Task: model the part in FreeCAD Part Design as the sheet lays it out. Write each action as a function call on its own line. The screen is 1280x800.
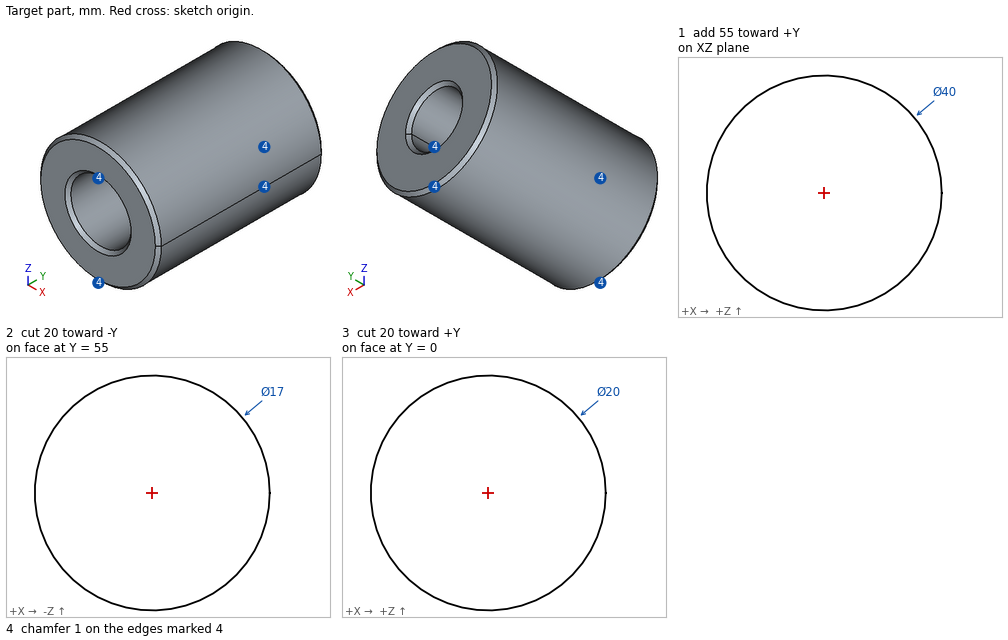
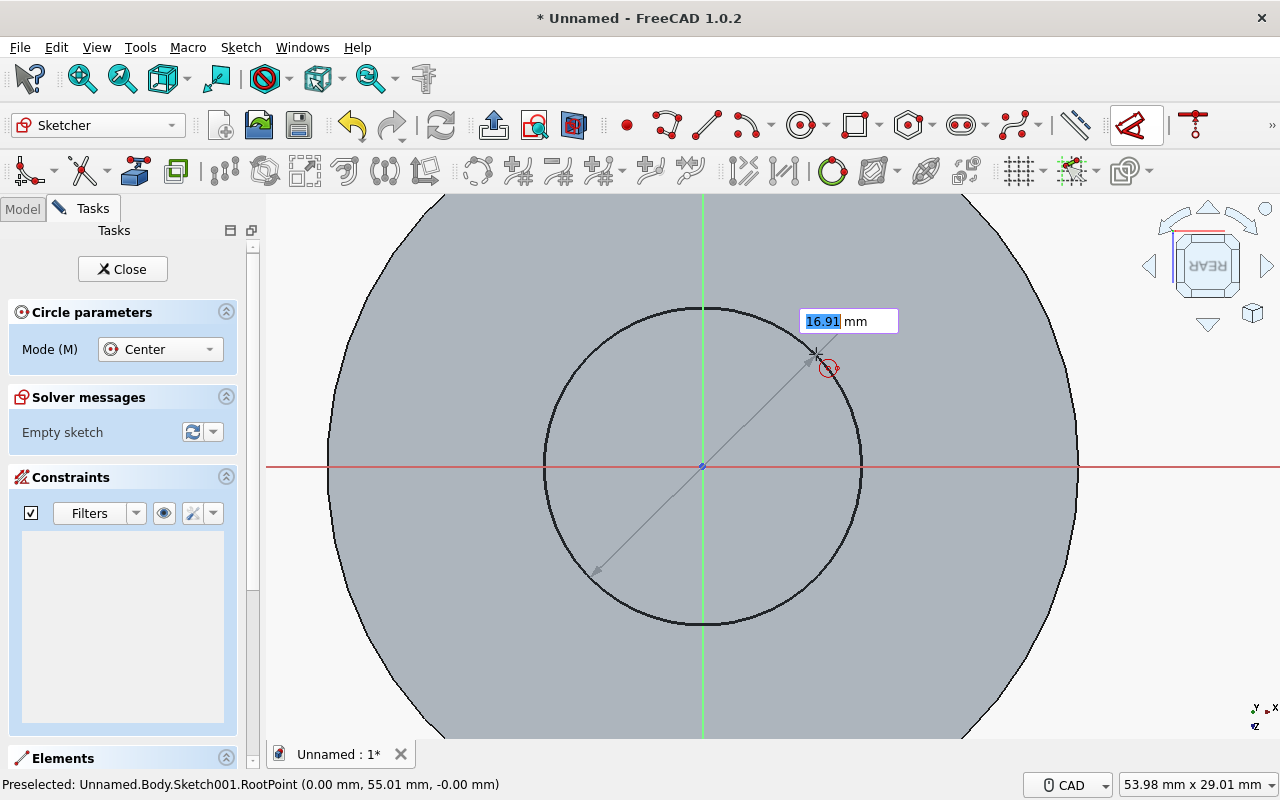
text(17)
key(Return)
key(Escape)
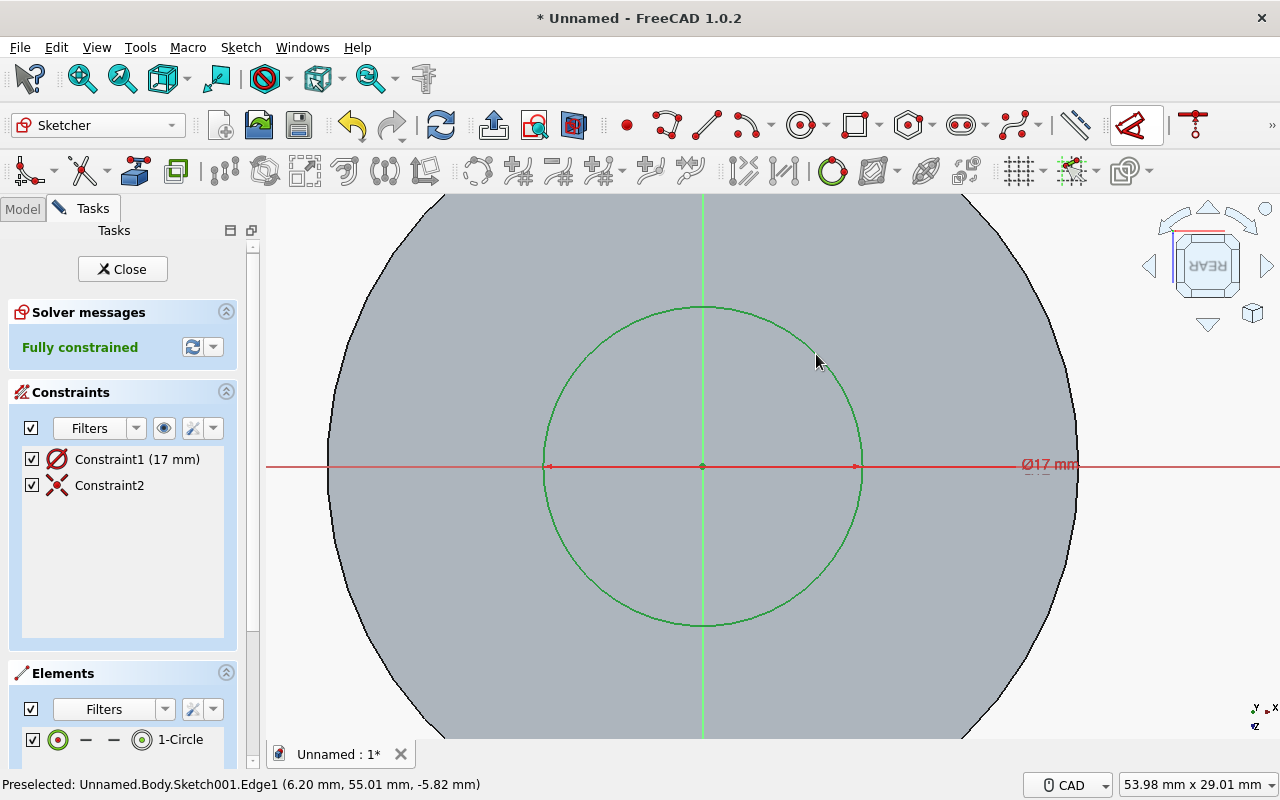
click(123, 269)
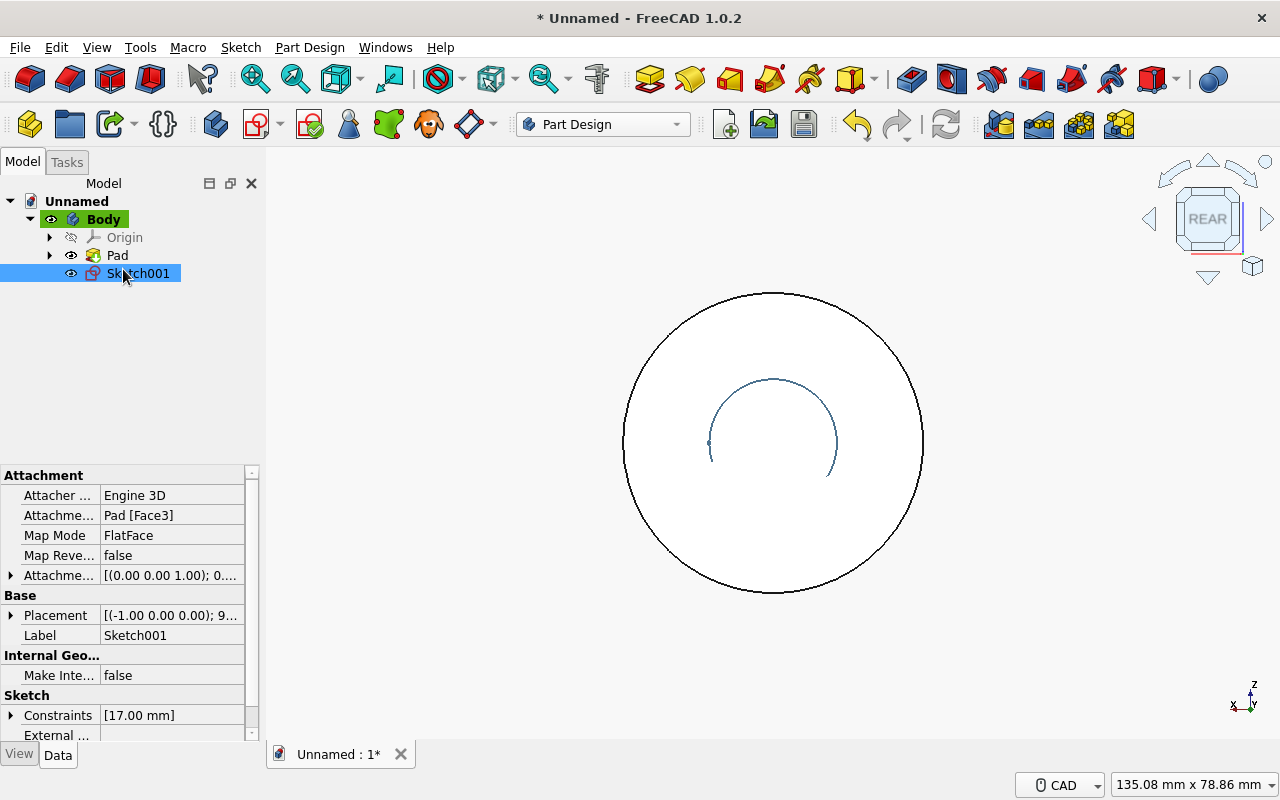
click(912, 80)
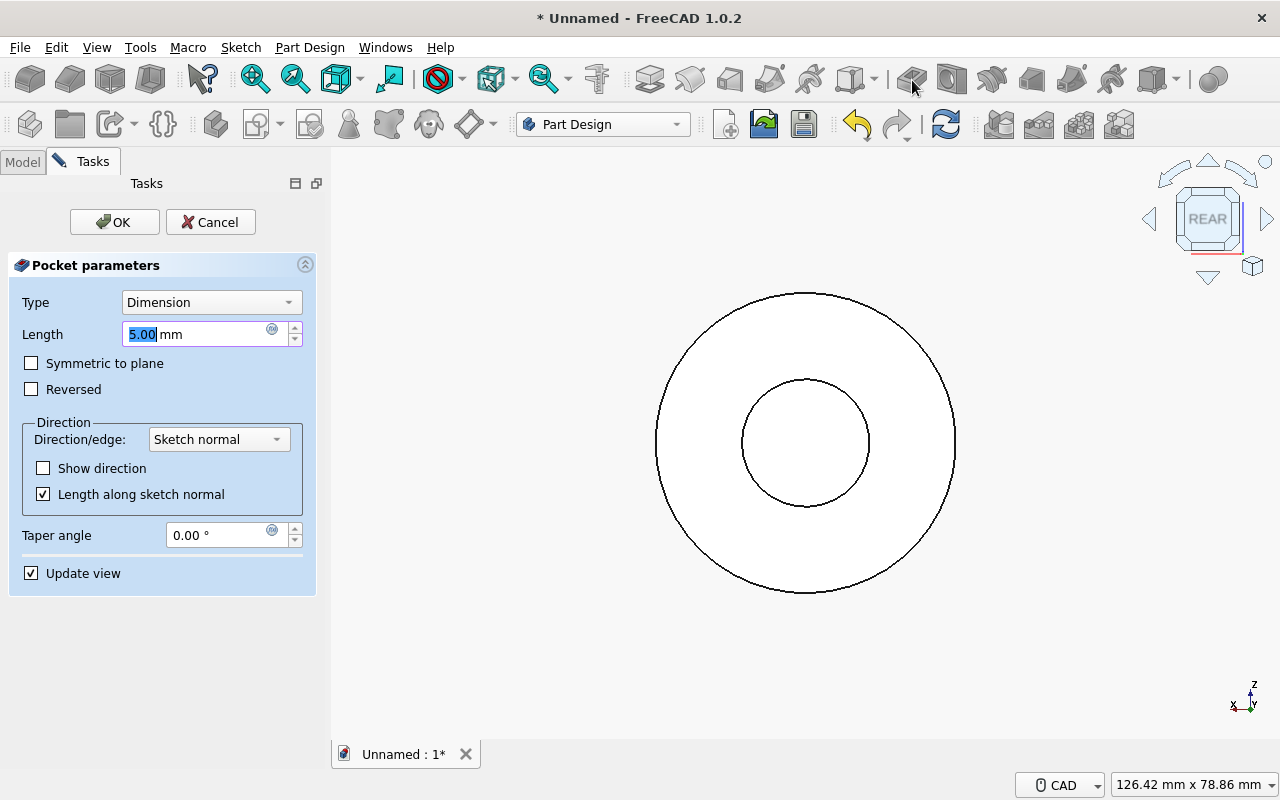
text(20)
key(Tab)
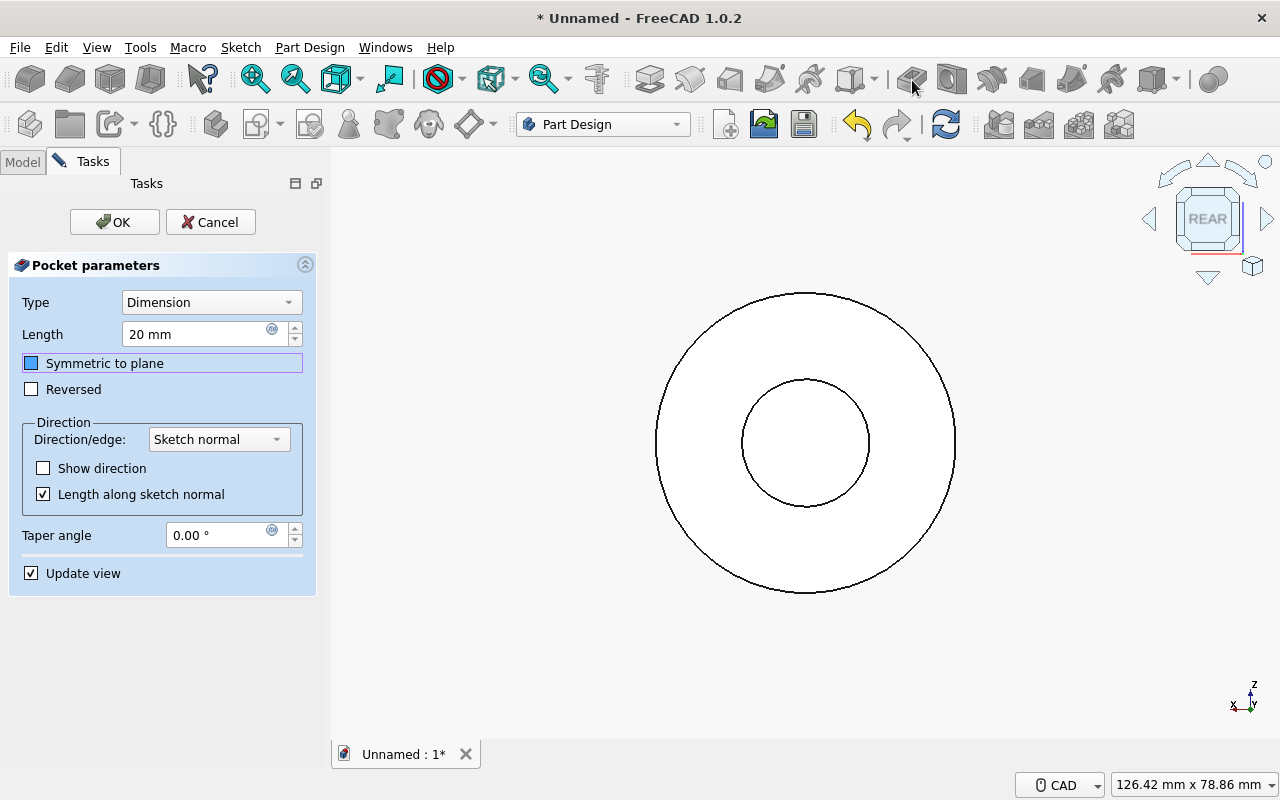
click(115, 222)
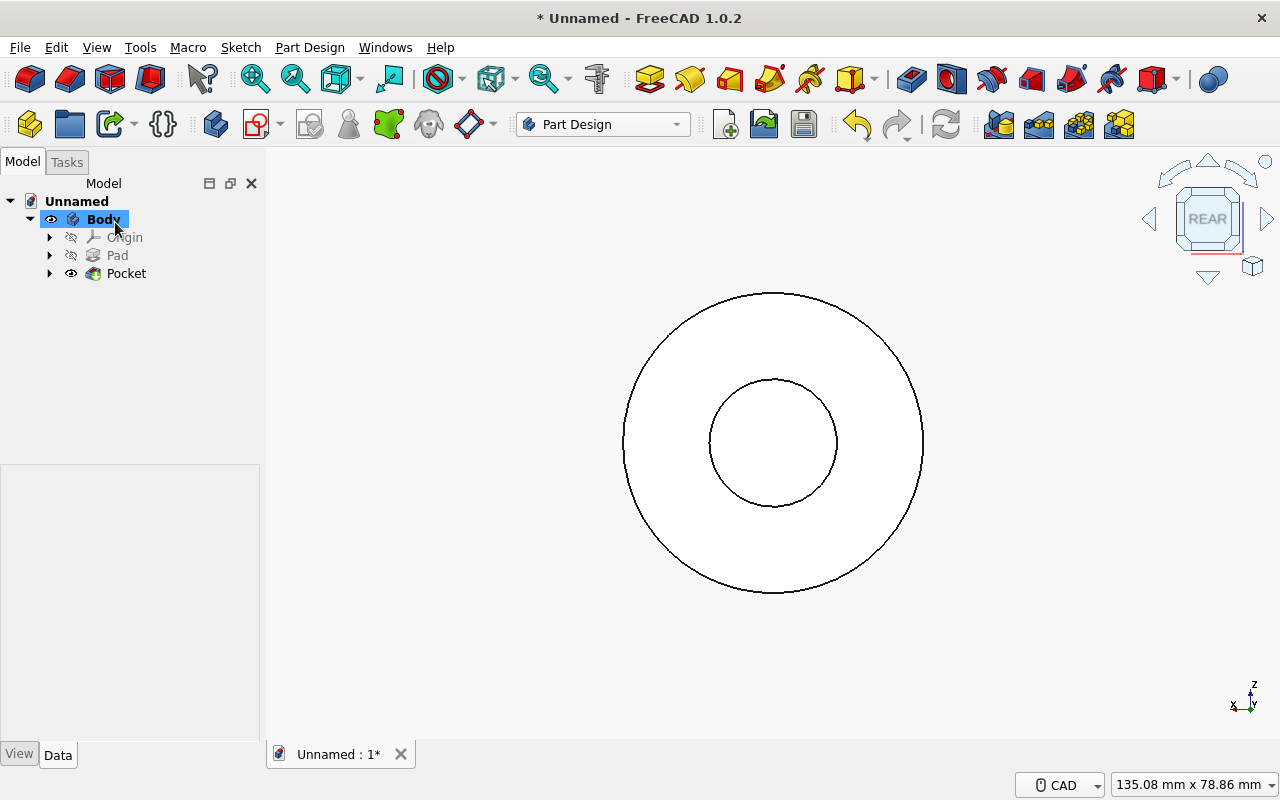
key(0)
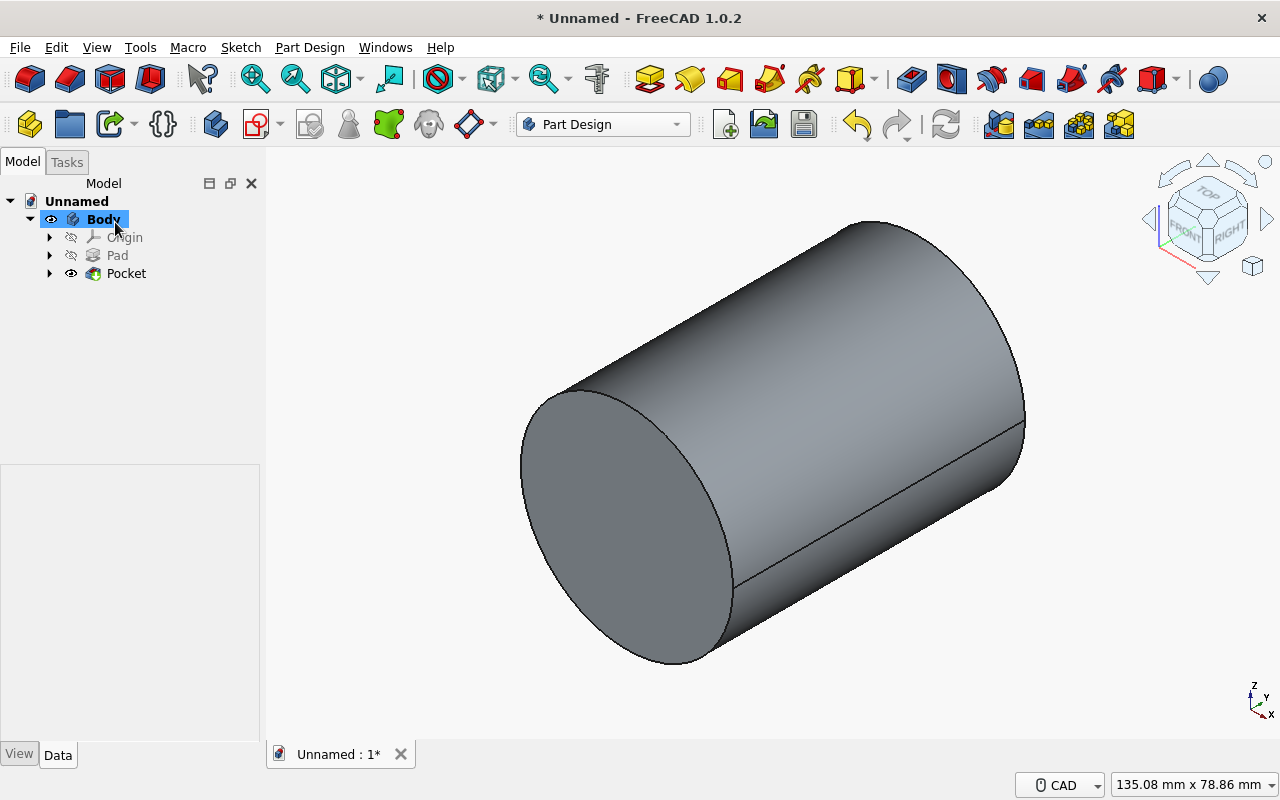
click(627, 526)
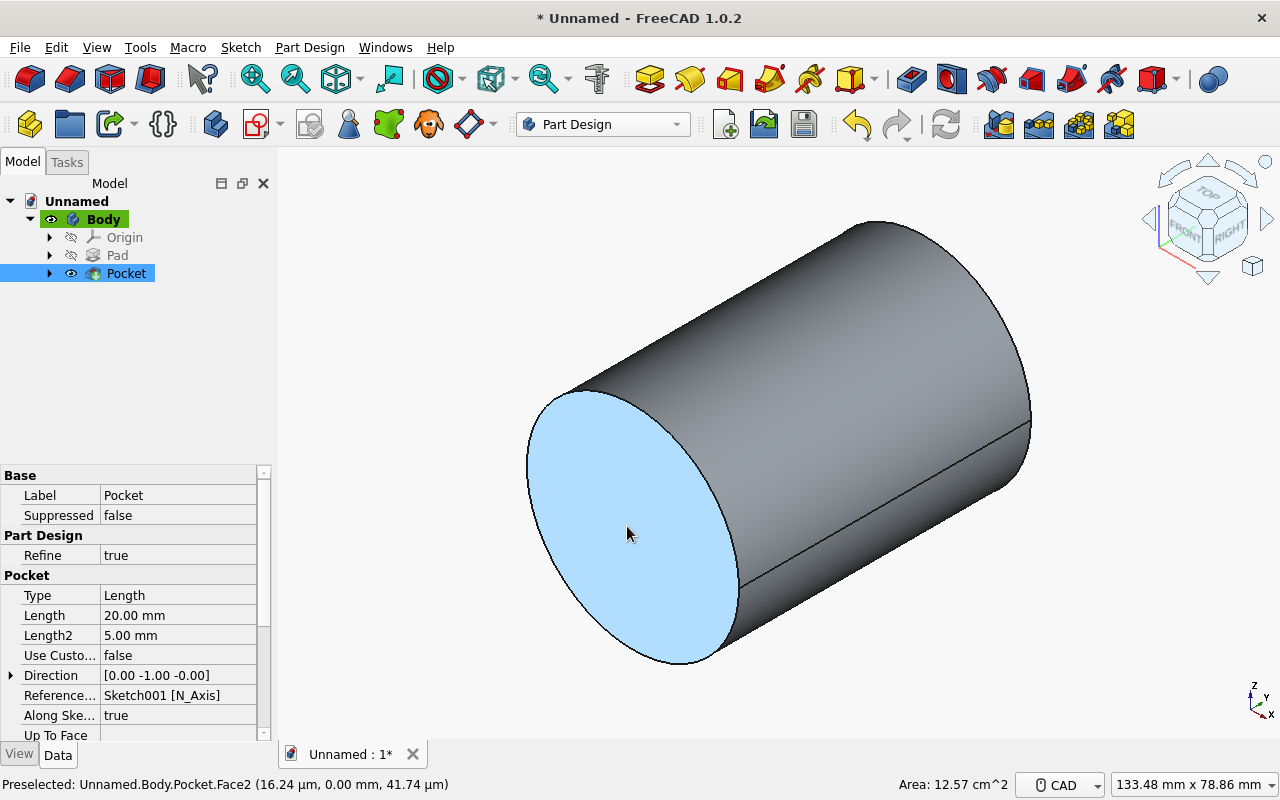
click(256, 124)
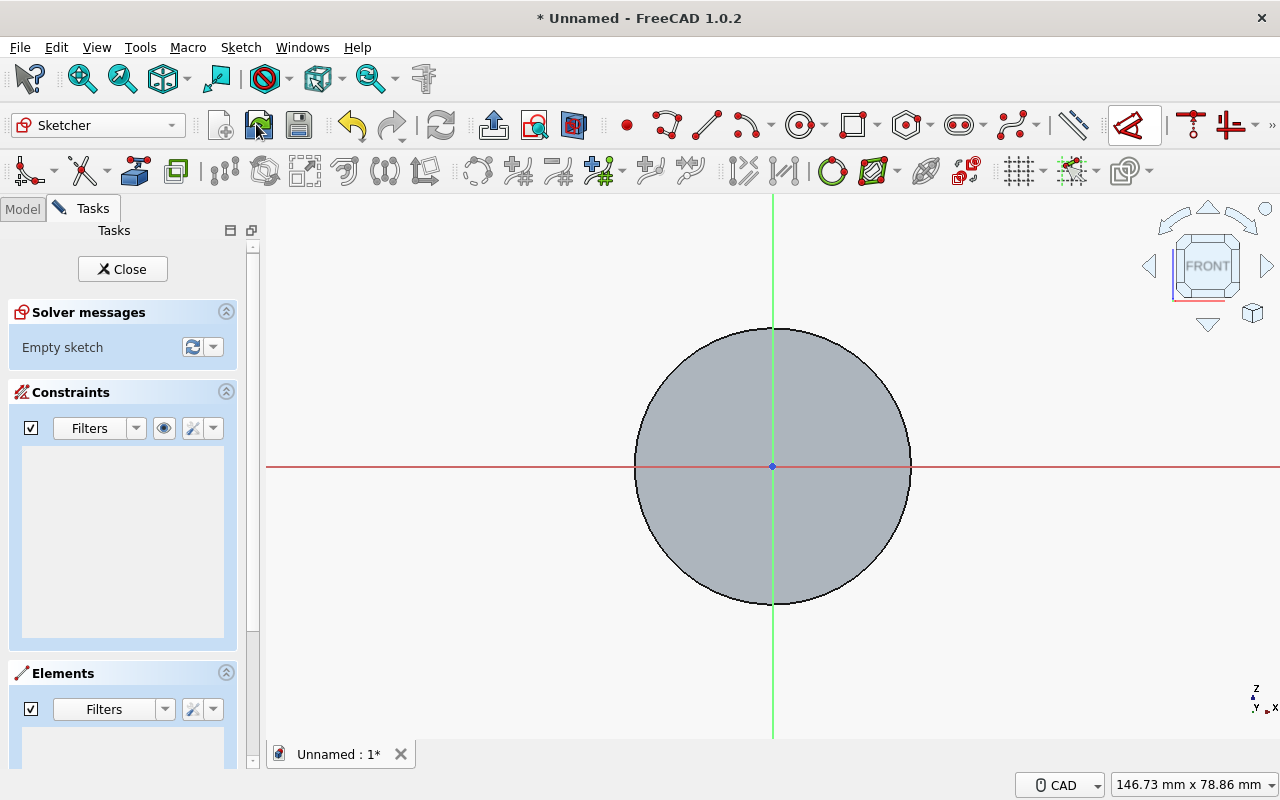
scroll(813, 467, up, 5)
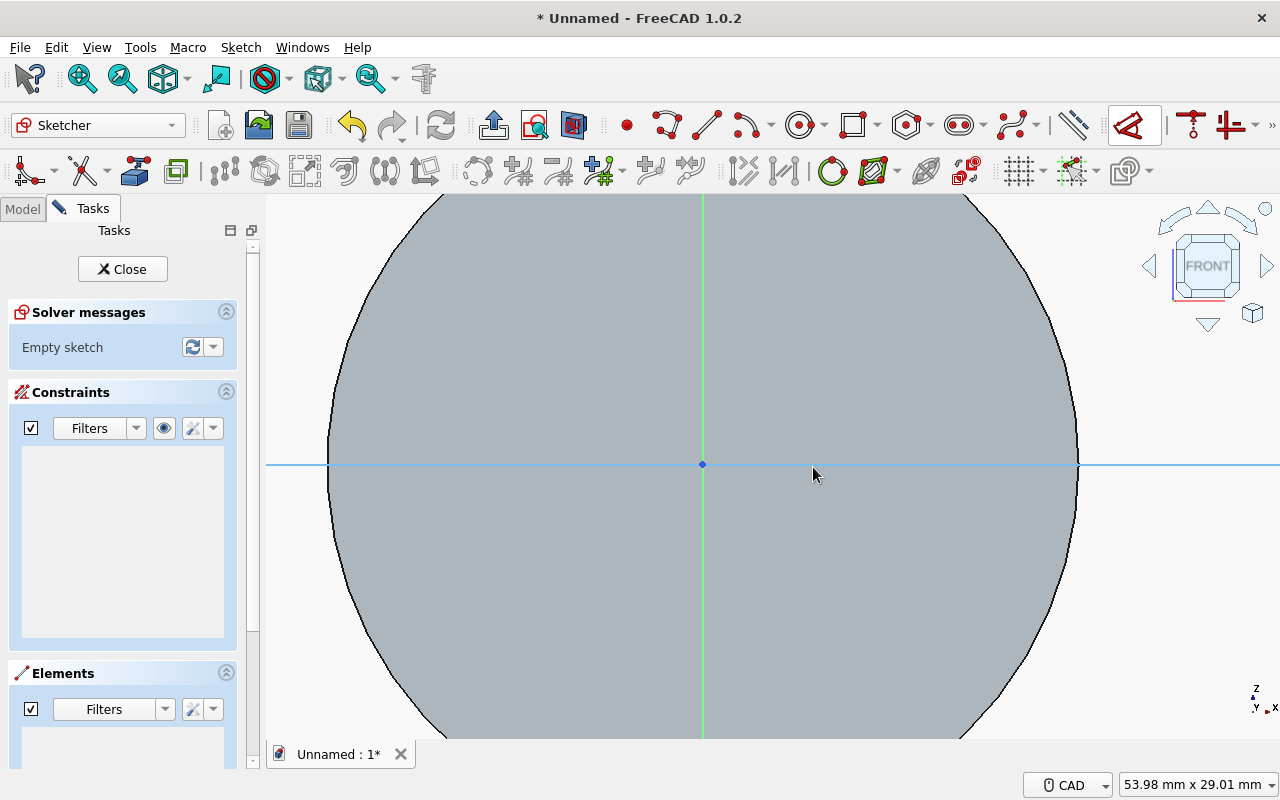
click(800, 126)